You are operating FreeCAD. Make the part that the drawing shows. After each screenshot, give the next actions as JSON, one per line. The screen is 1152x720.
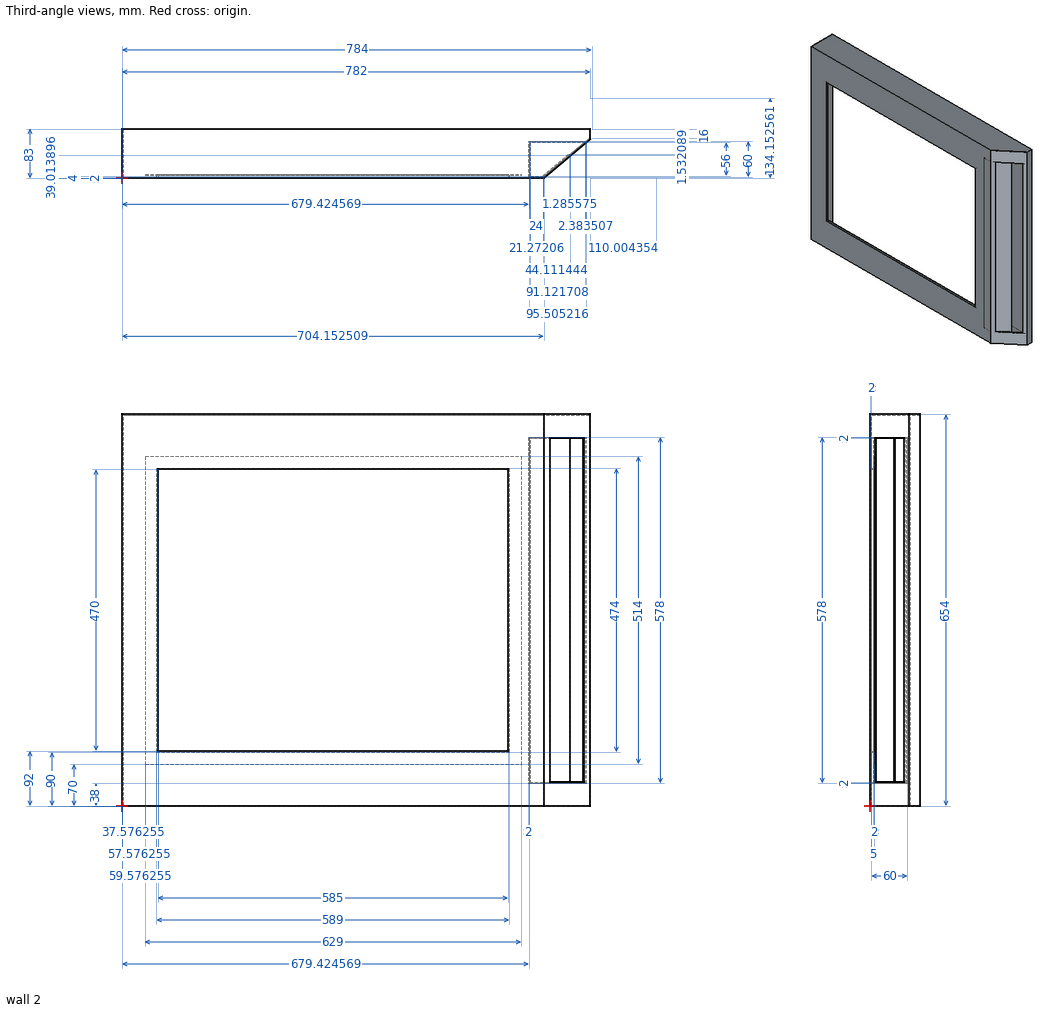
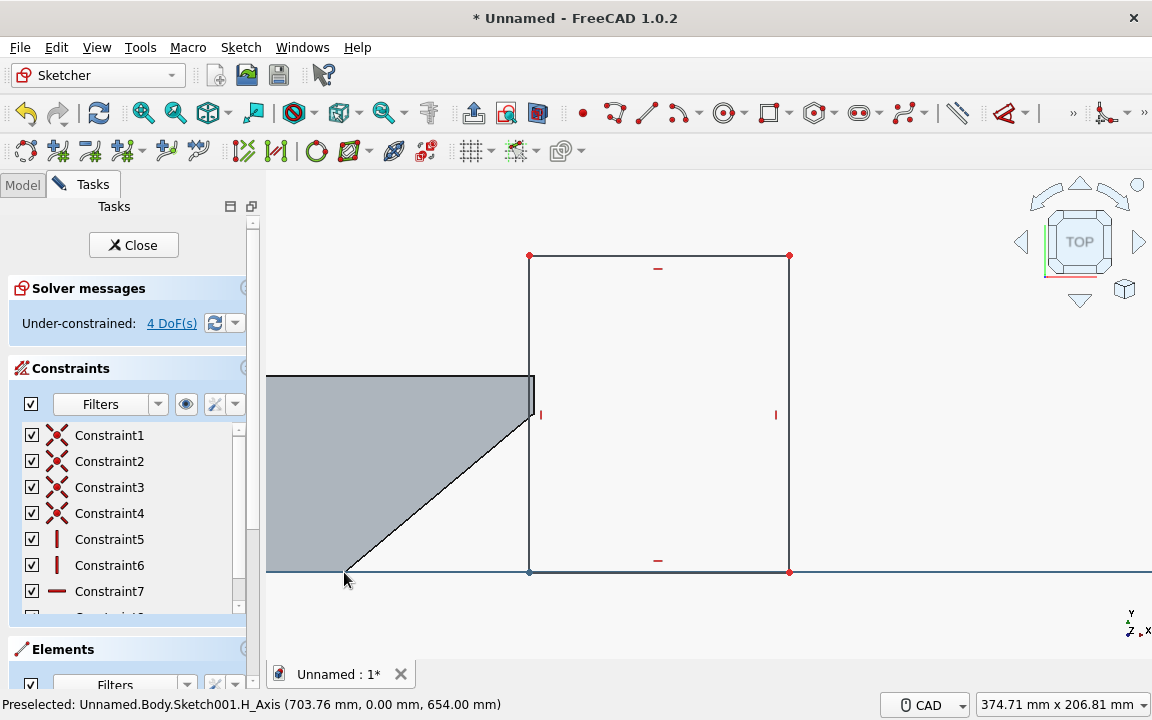
{"action": "key", "text": "c"}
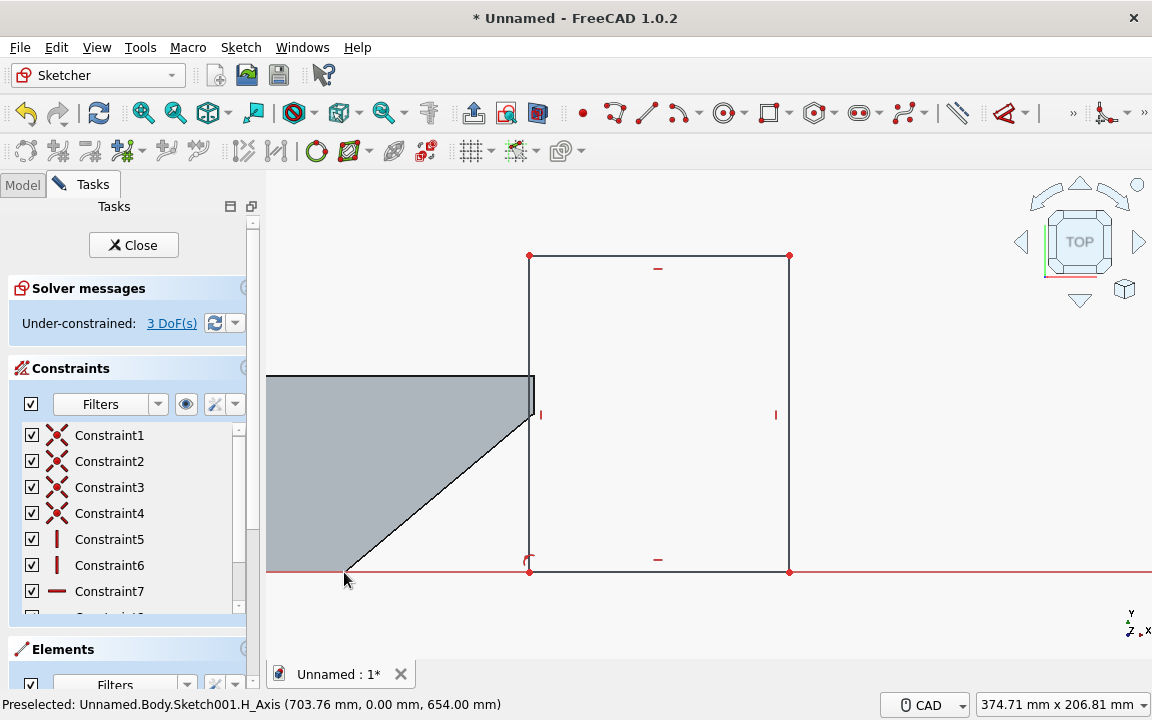
{"action": "key", "text": "d"}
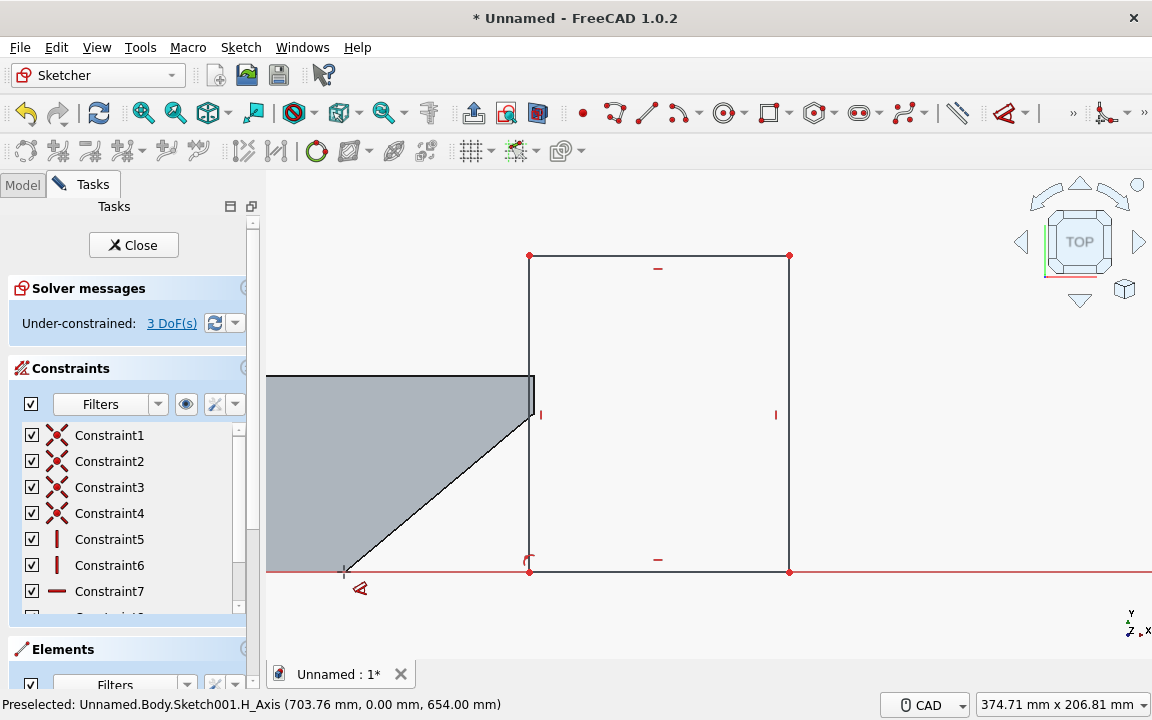
{"action": "left_click", "coordinate": [529, 256]}
{"action": "left_click", "coordinate": [412, 606]}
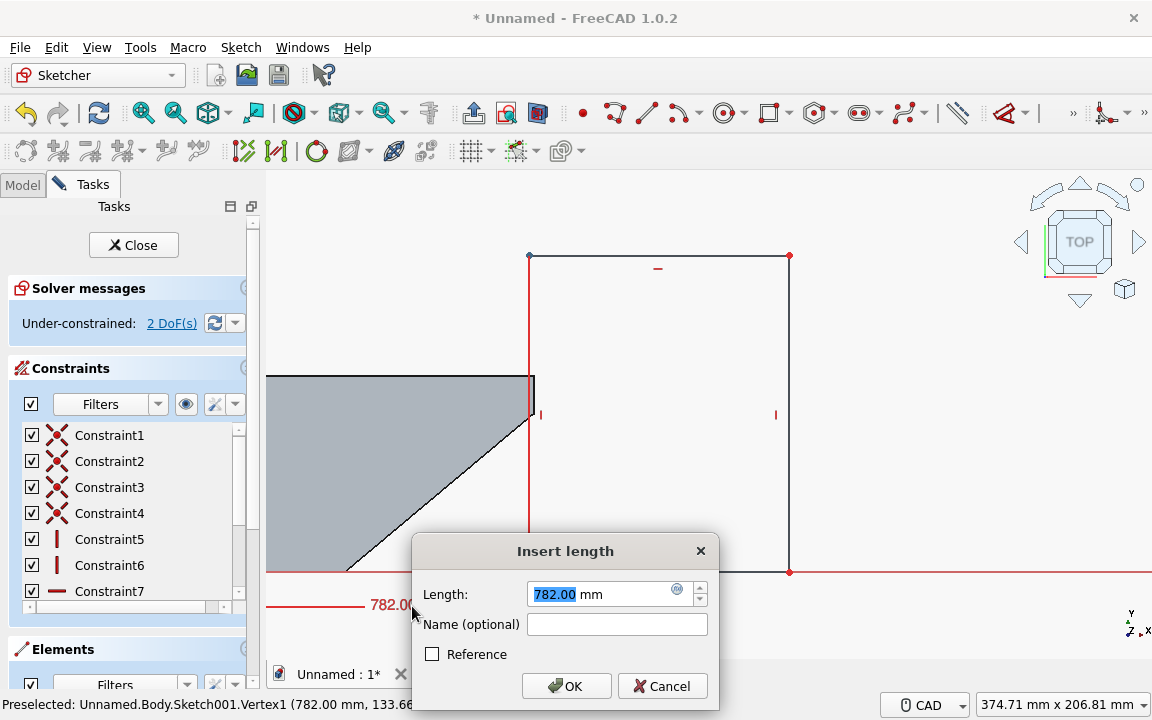
{"action": "type", "text": "782"}
{"action": "key", "text": "Return"}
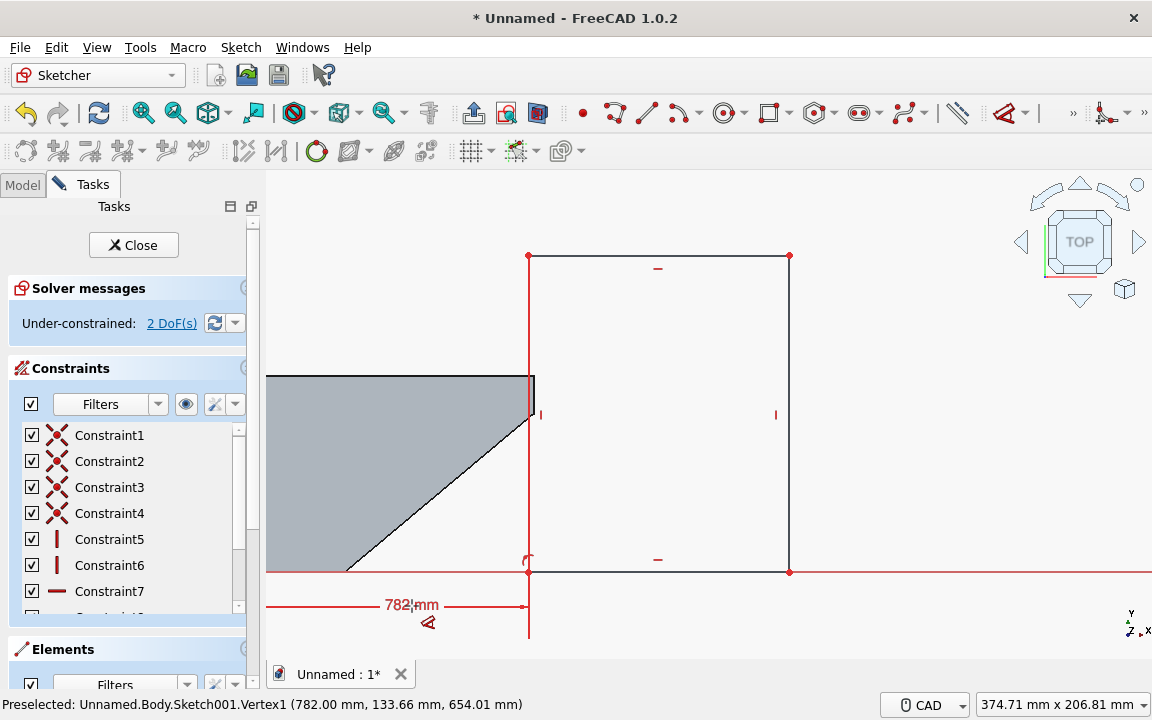
{"action": "left_click", "coordinate": [529, 351]}
{"action": "left_click", "coordinate": [495, 414]}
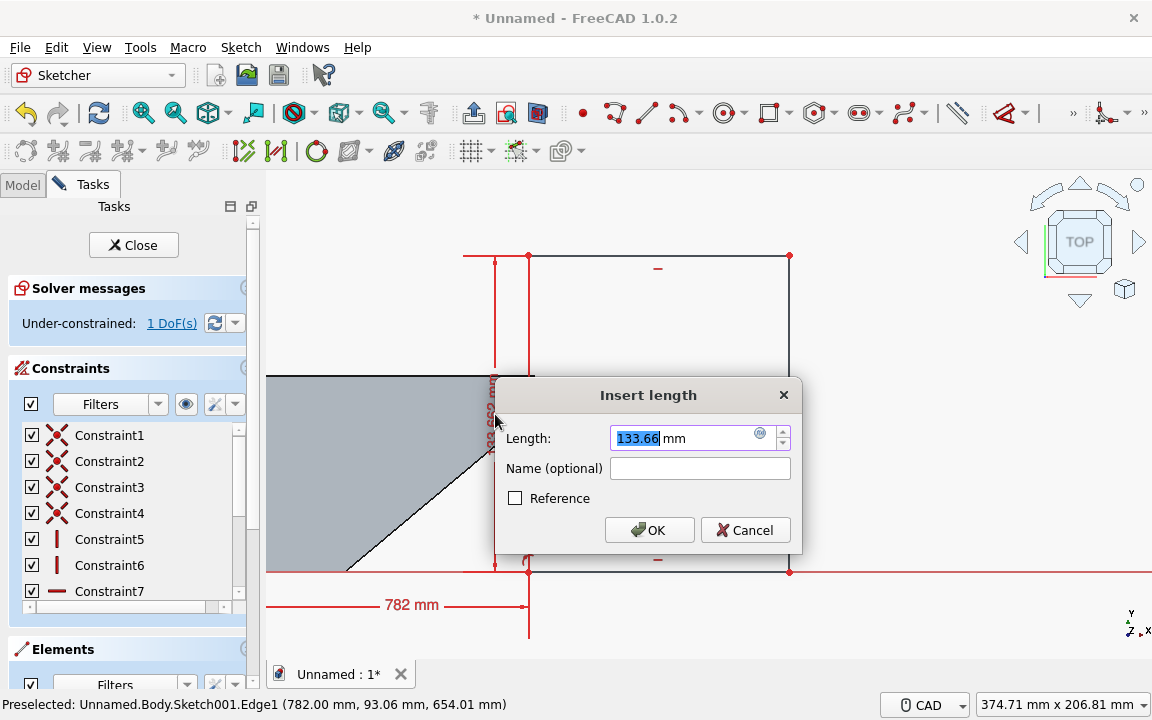
{"action": "type", "text": "134.152561"}
{"action": "key", "text": "Return"}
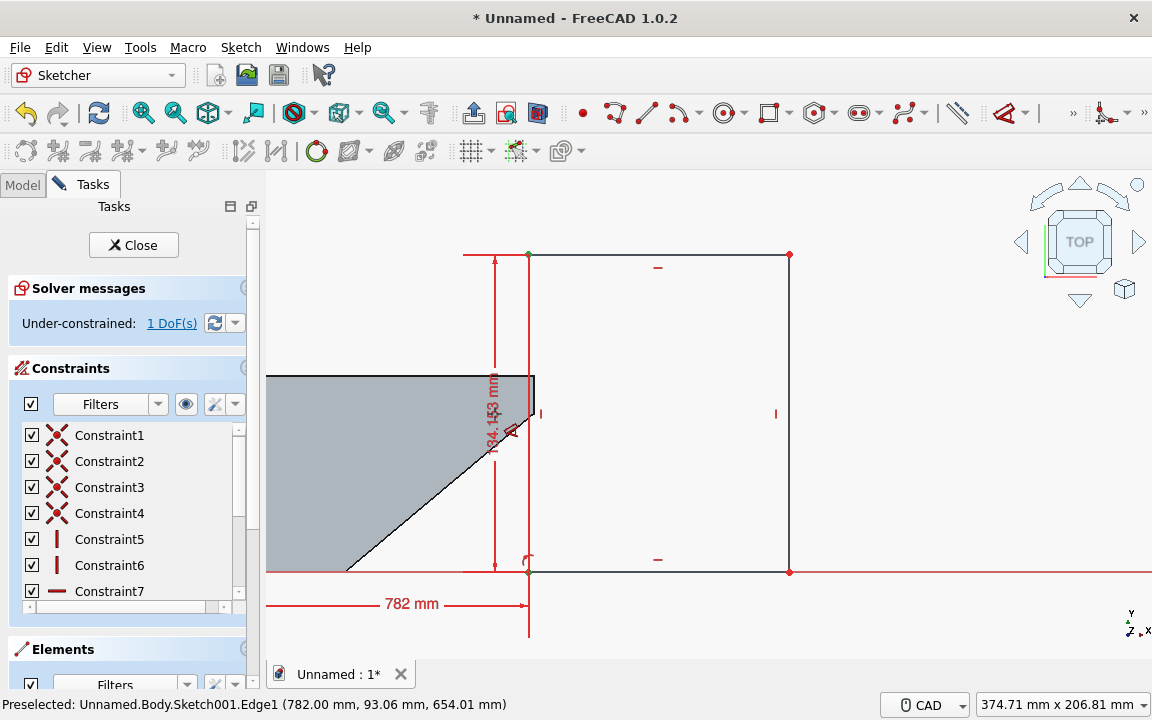
{"action": "left_click", "coordinate": [607, 572]}
{"action": "left_click", "coordinate": [659, 606]}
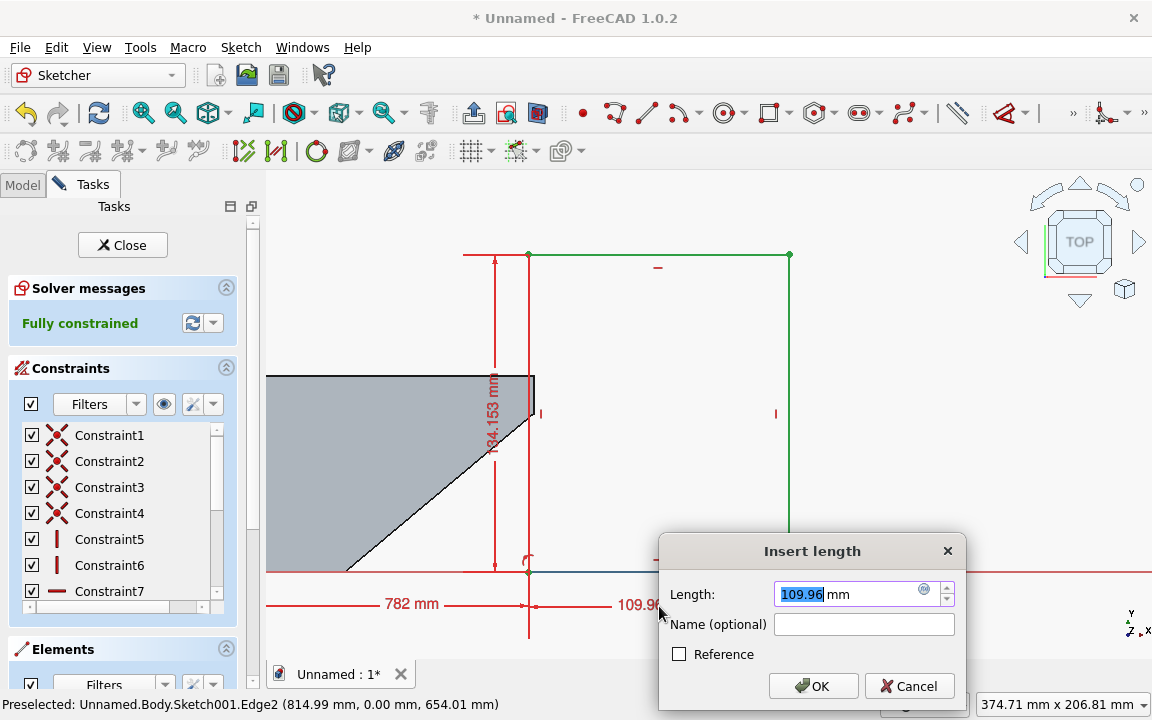
{"action": "type", "text": "110.004354"}
{"action": "key", "text": "Return"}
{"action": "key", "text": "Escape"}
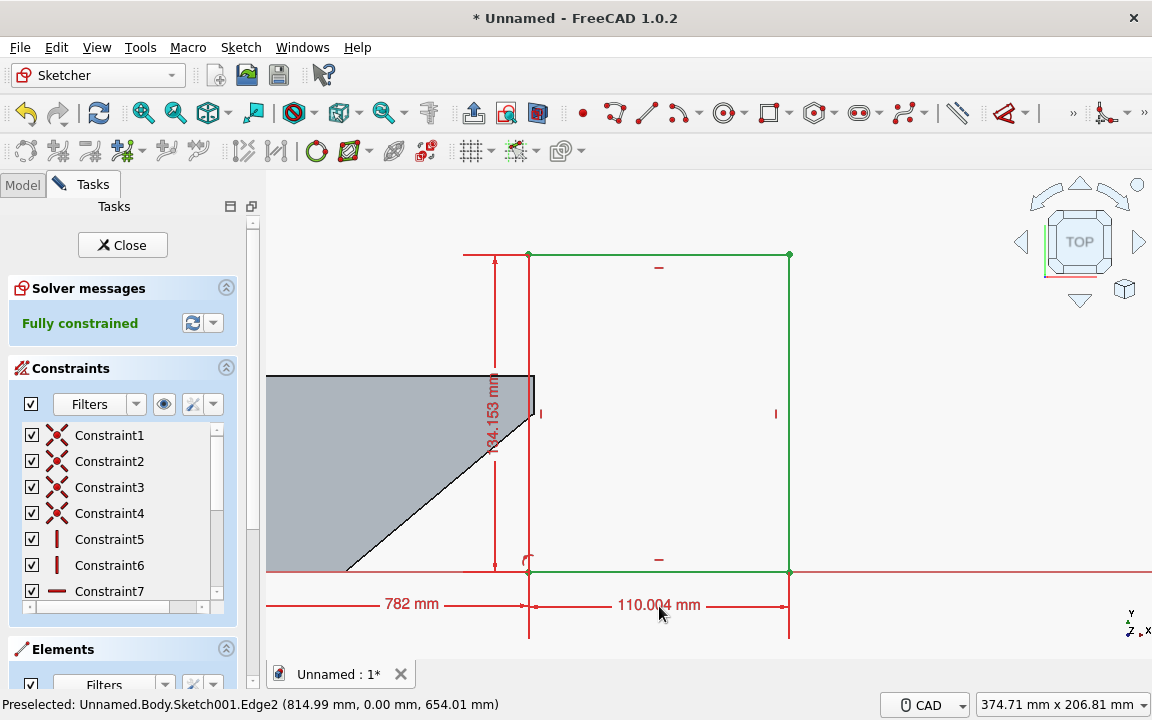
{"action": "left_click", "coordinate": [123, 245]}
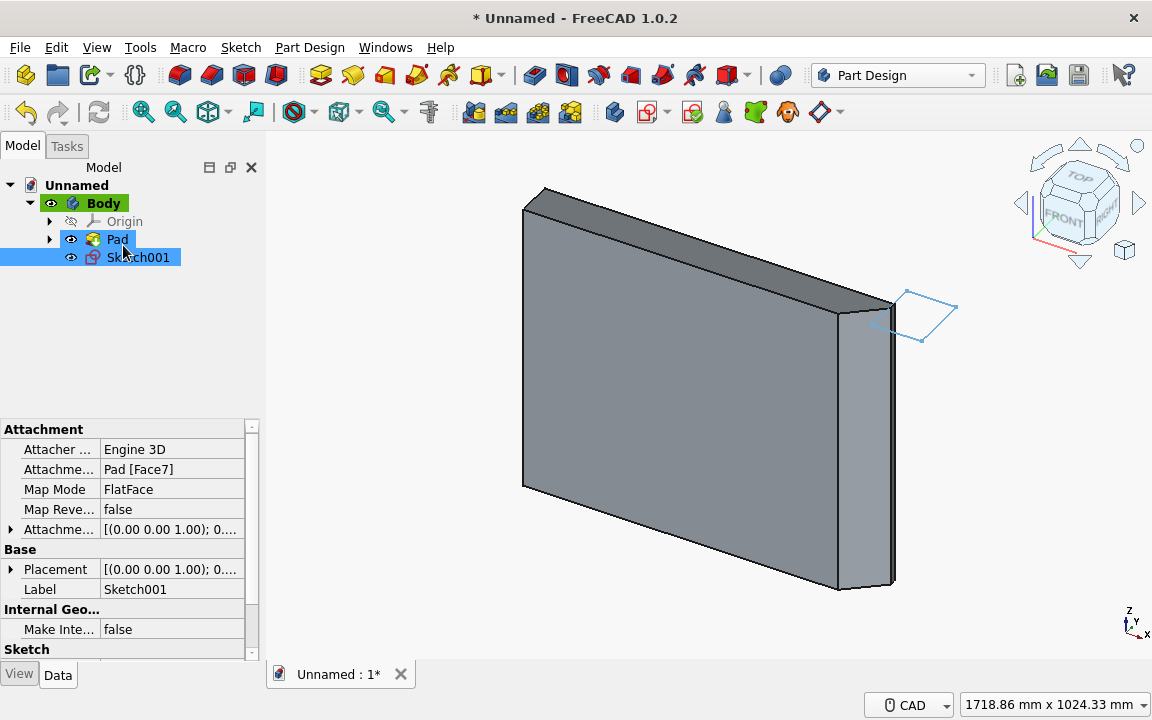
{"action": "left_click", "coordinate": [536, 76]}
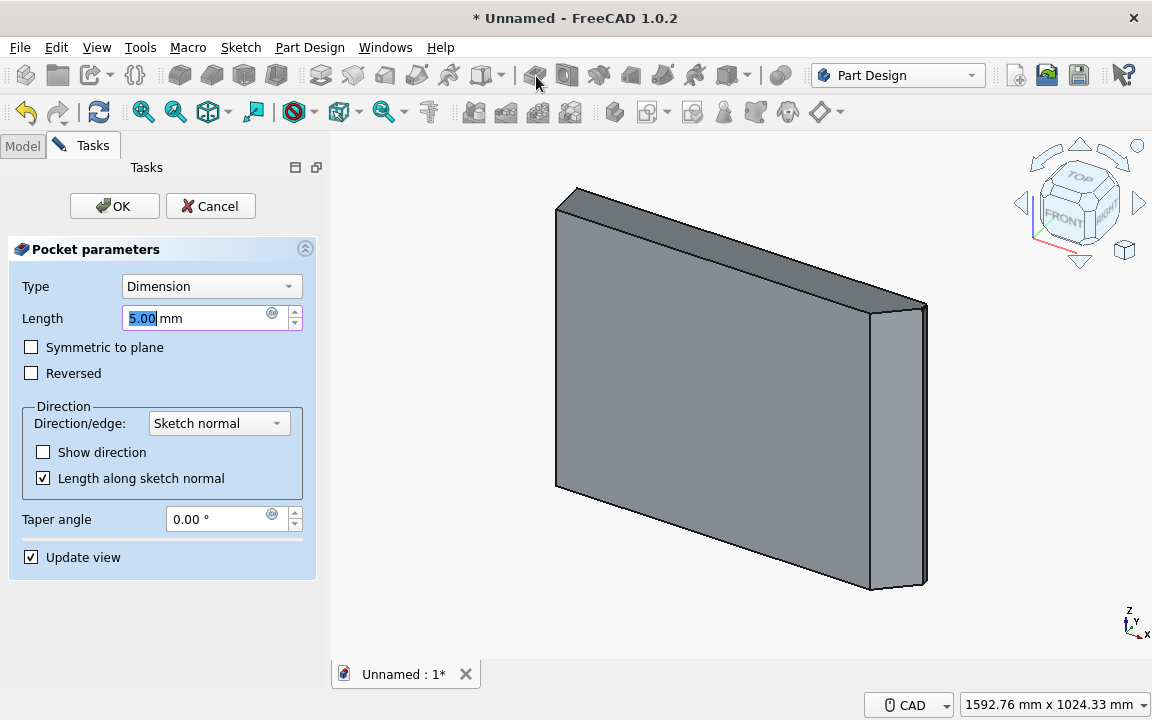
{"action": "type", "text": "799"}
{"action": "key", "text": "Tab"}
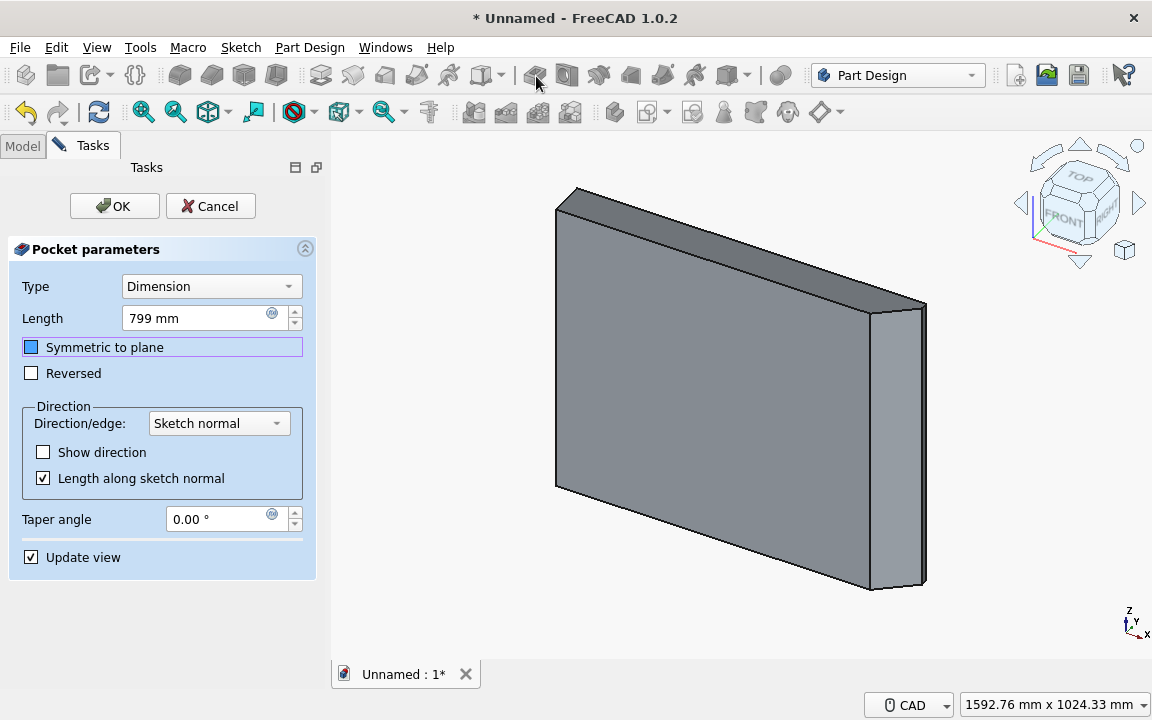
{"action": "left_click", "coordinate": [115, 206]}